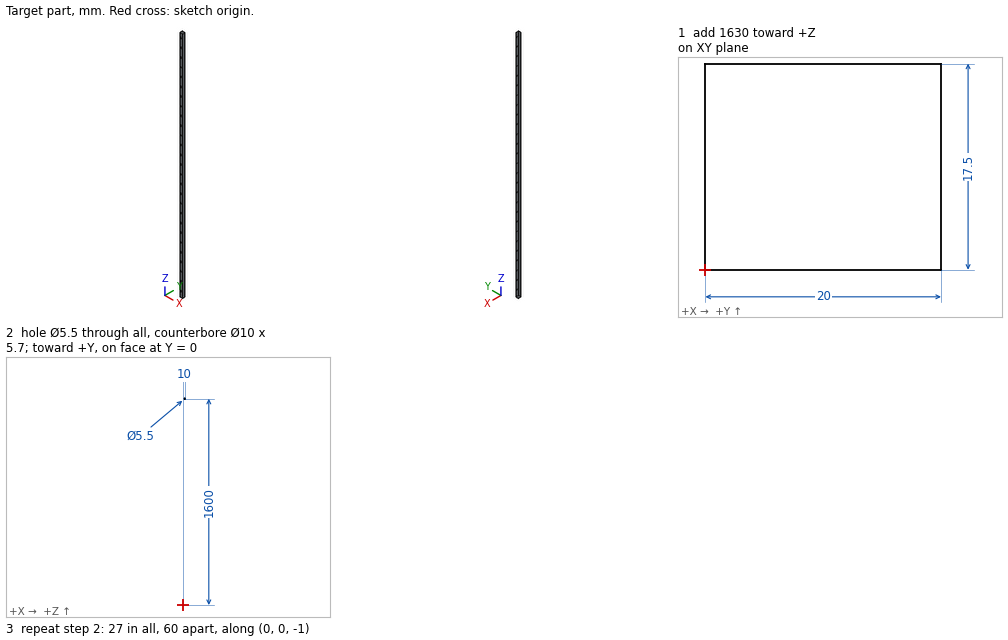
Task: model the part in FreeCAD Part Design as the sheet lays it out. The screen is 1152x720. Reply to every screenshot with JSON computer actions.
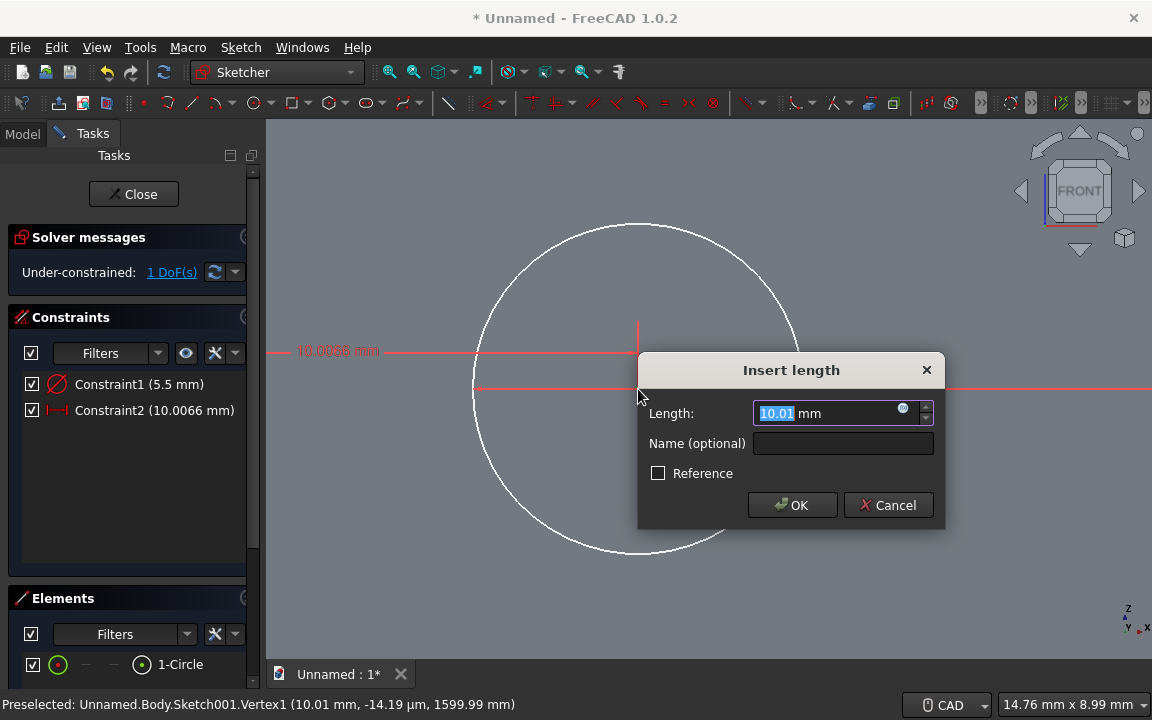
{"action": "type", "text": "10"}
{"action": "key", "text": "Return"}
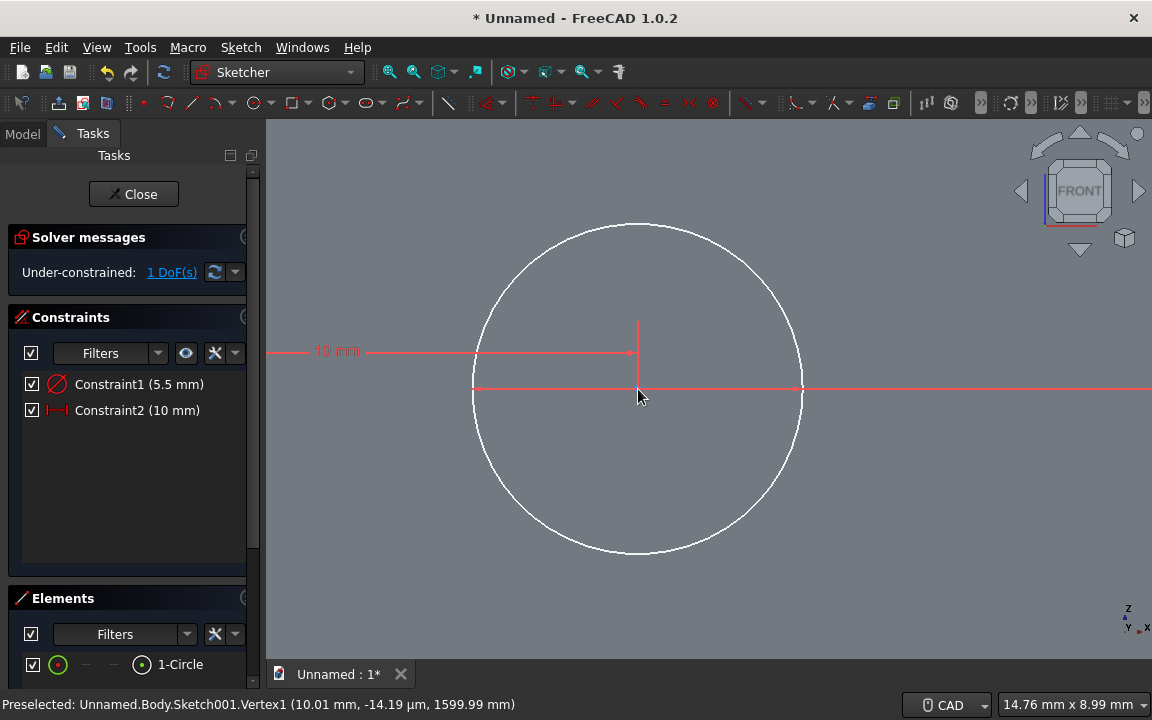
{"action": "left_click", "coordinate": [638, 389]}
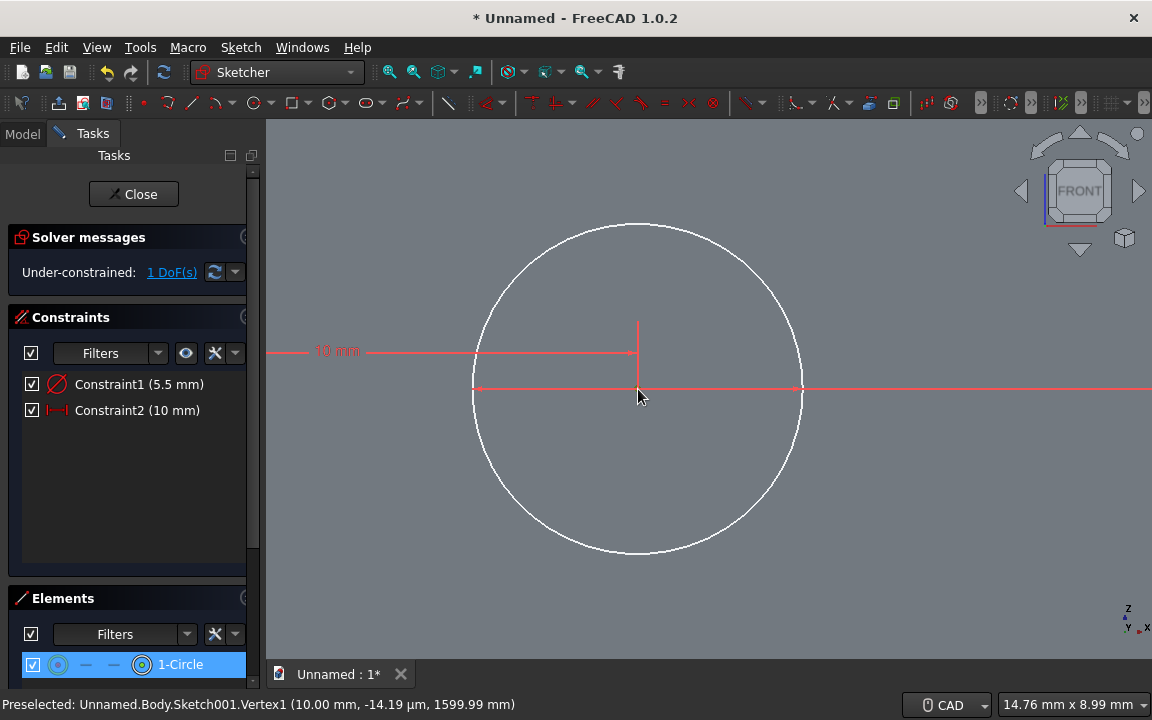
{"action": "left_click", "coordinate": [504, 104]}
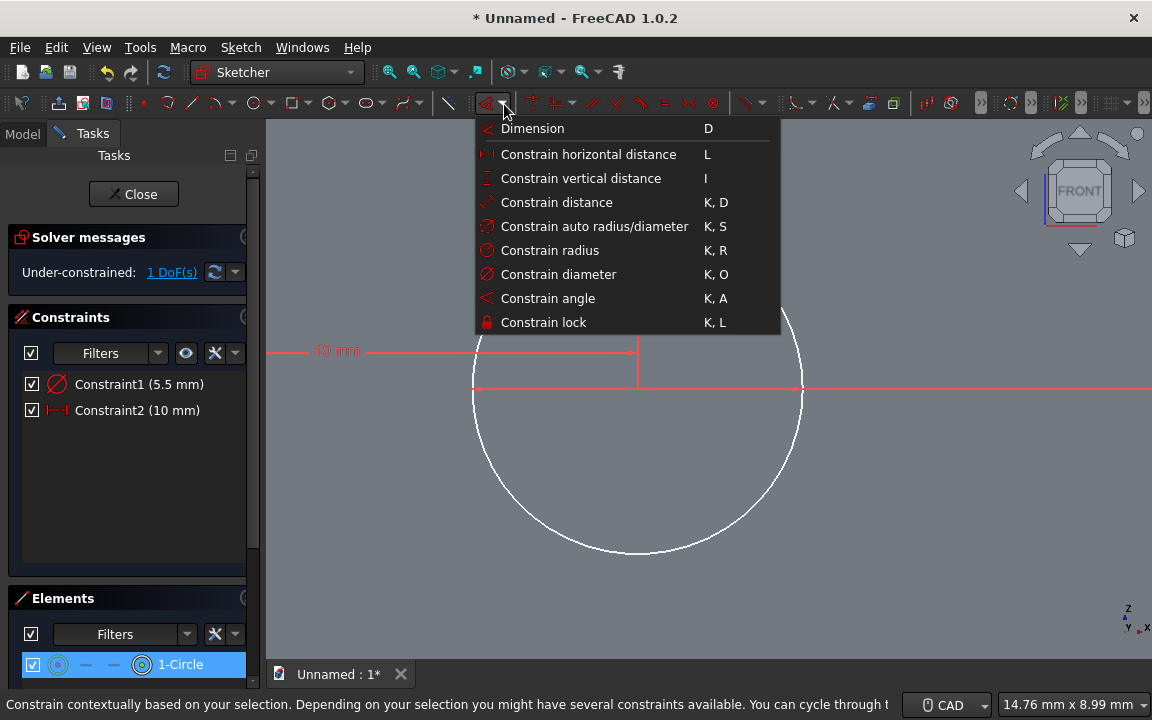
{"action": "left_click", "coordinate": [628, 178]}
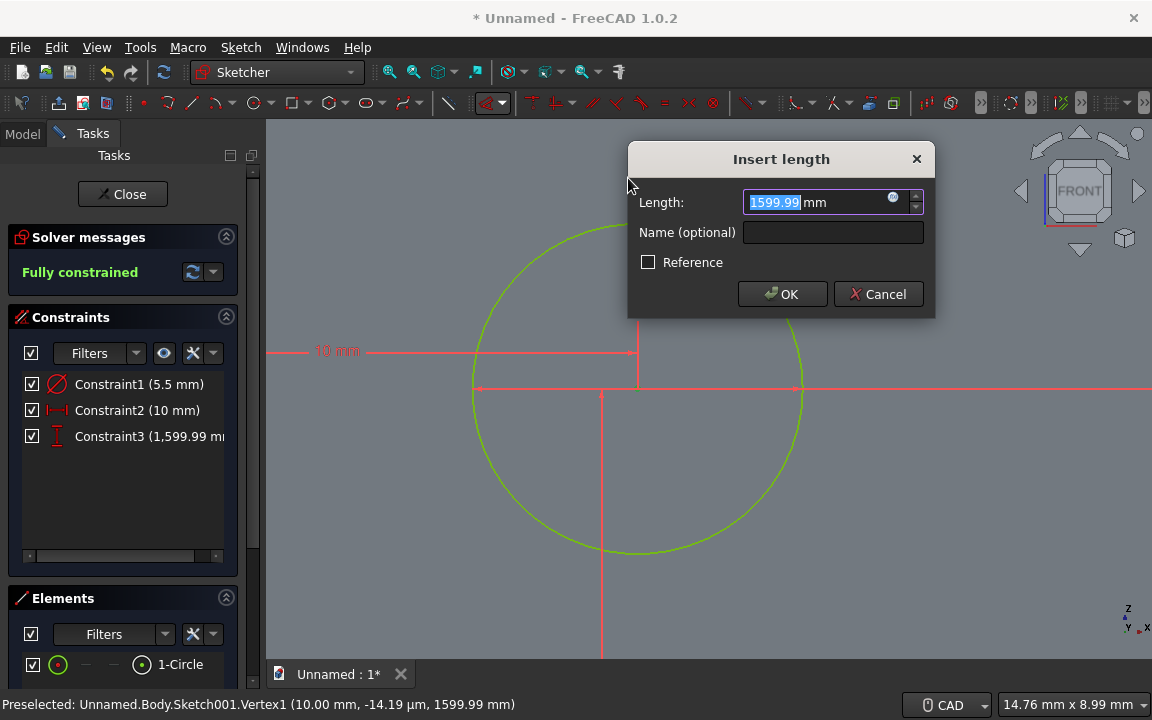
{"action": "type", "text": "1600"}
{"action": "key", "text": "Return"}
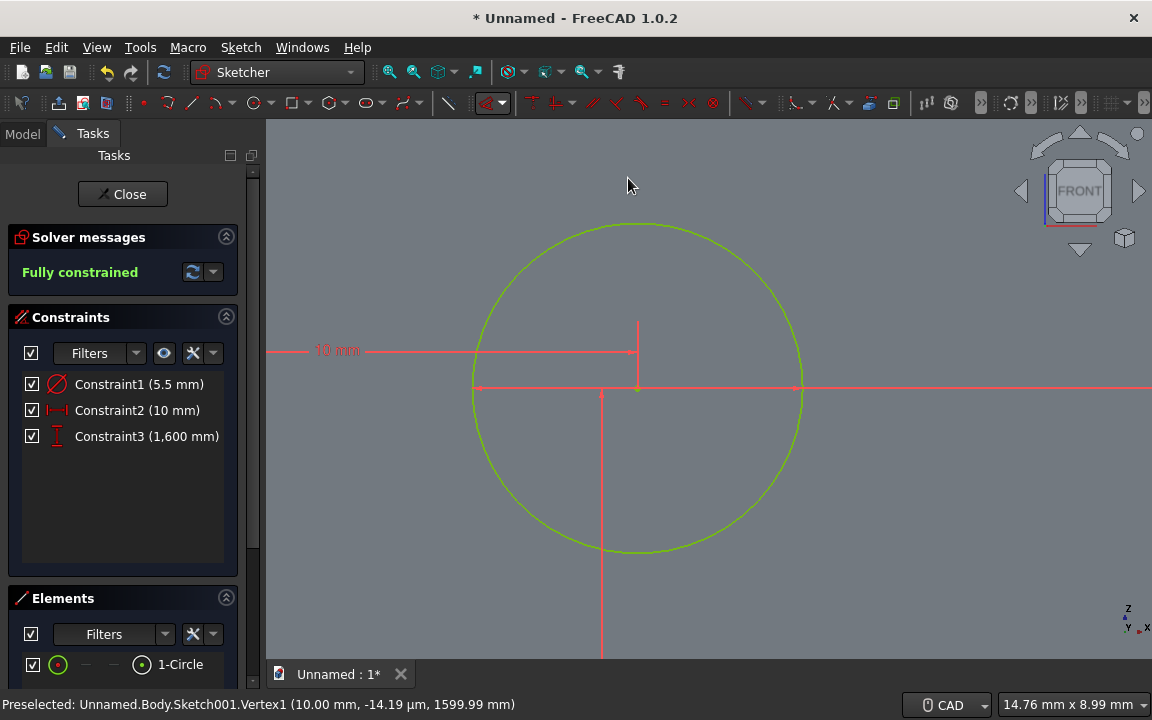
{"action": "left_click", "coordinate": [123, 194]}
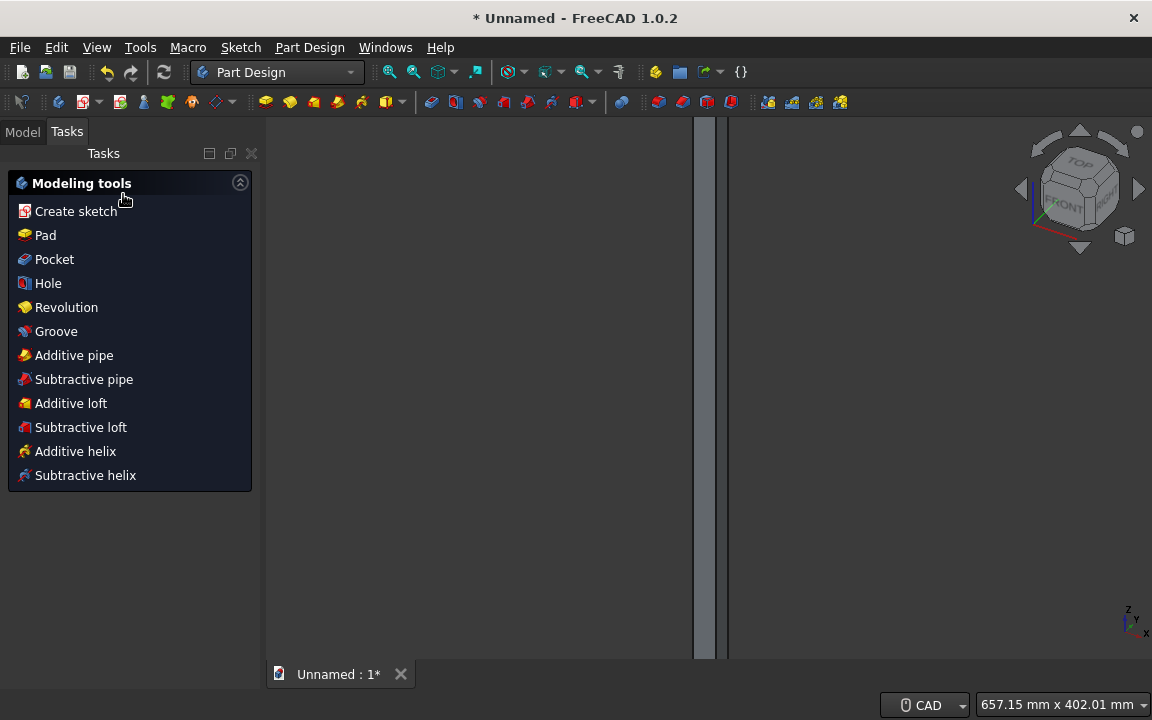
{"action": "left_click", "coordinate": [456, 102]}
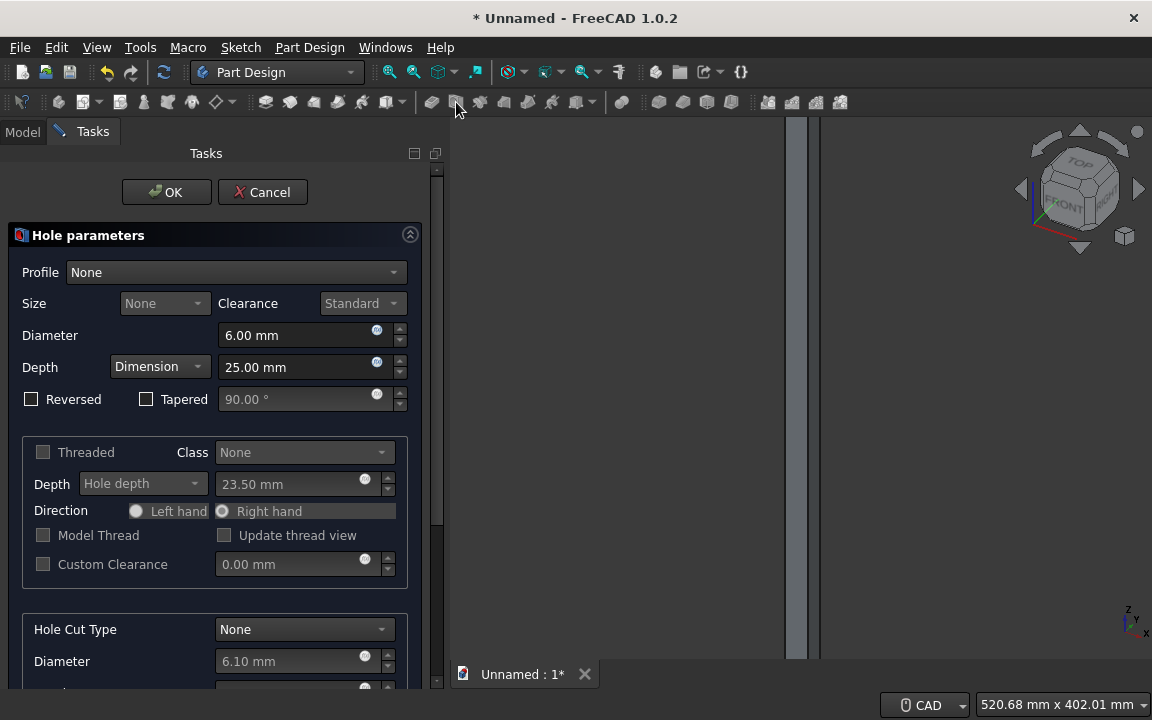
{"action": "triple_click", "coordinate": [305, 335]}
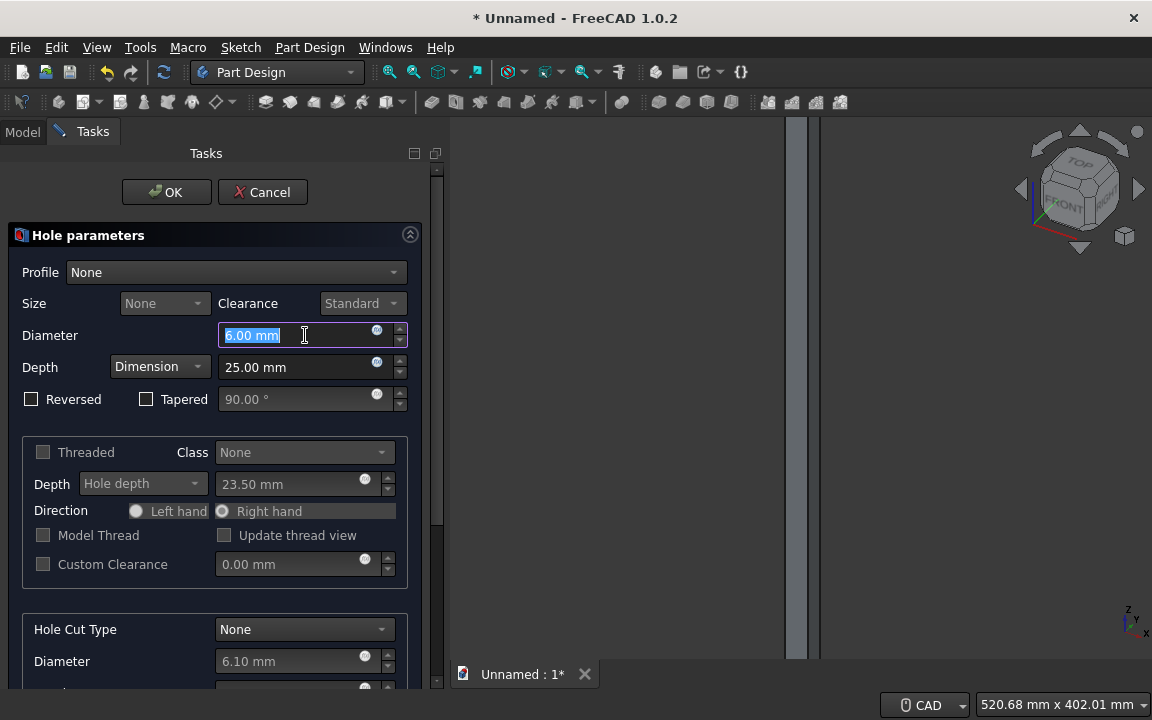
{"action": "type", "text": "5.5"}
{"action": "key", "text": "Tab"}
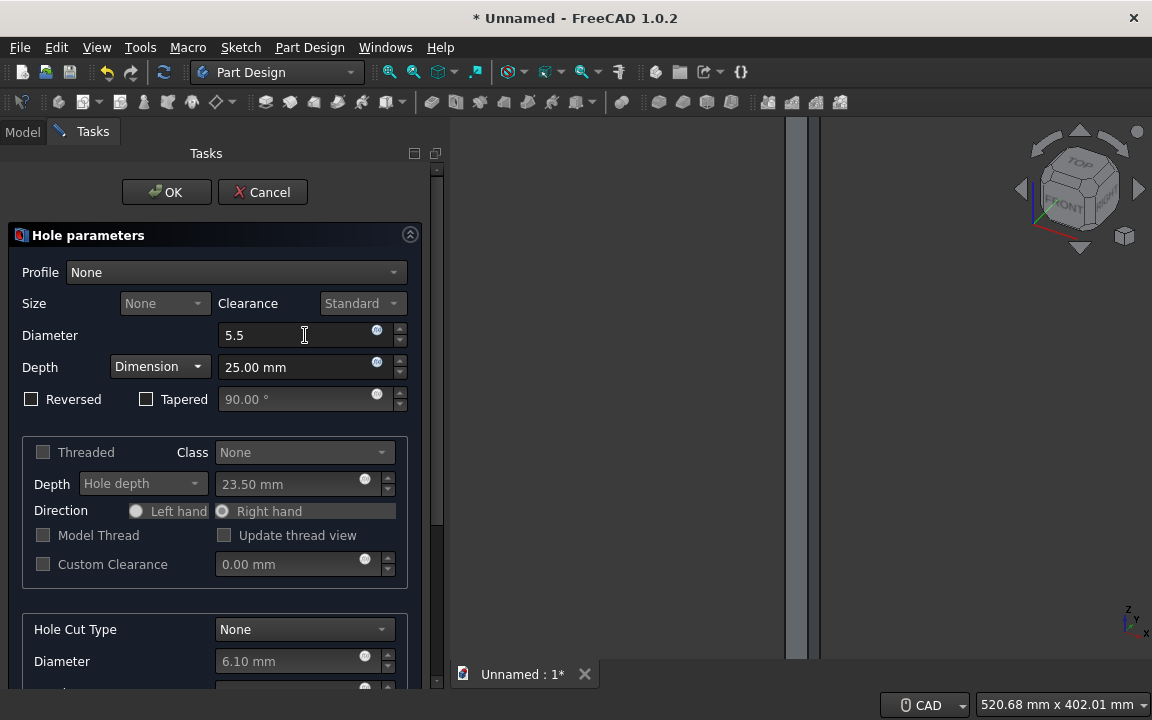
{"action": "left_click", "coordinate": [161, 366]}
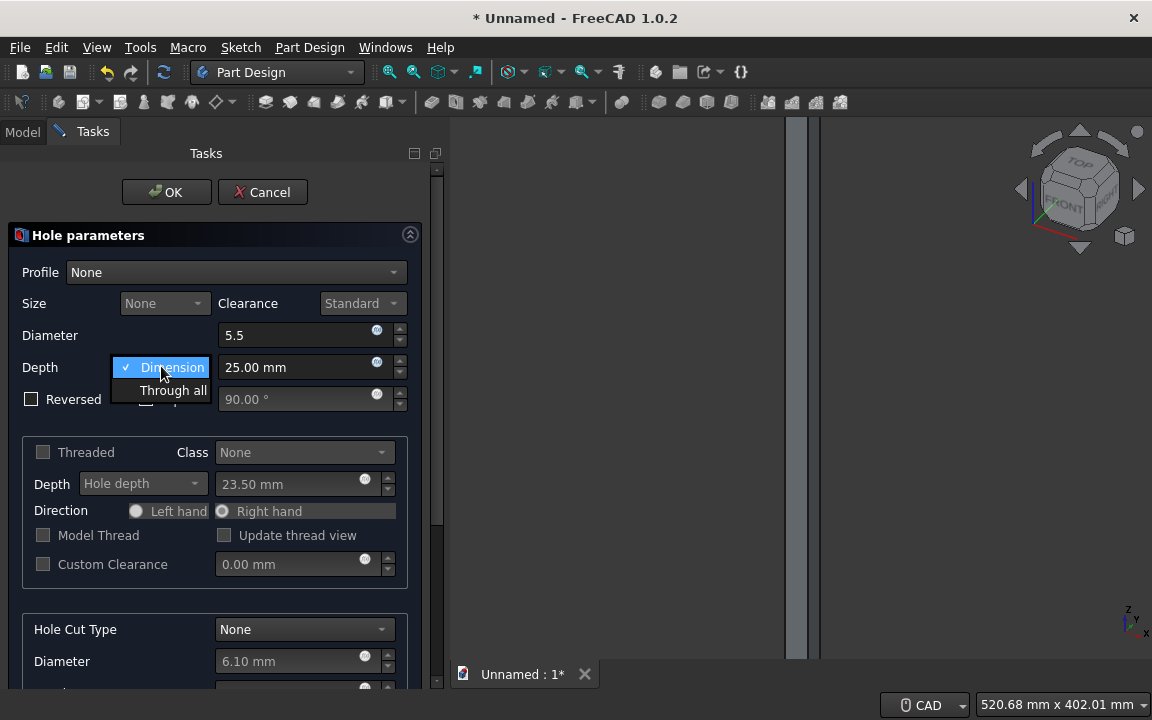
{"action": "left_click", "coordinate": [160, 390]}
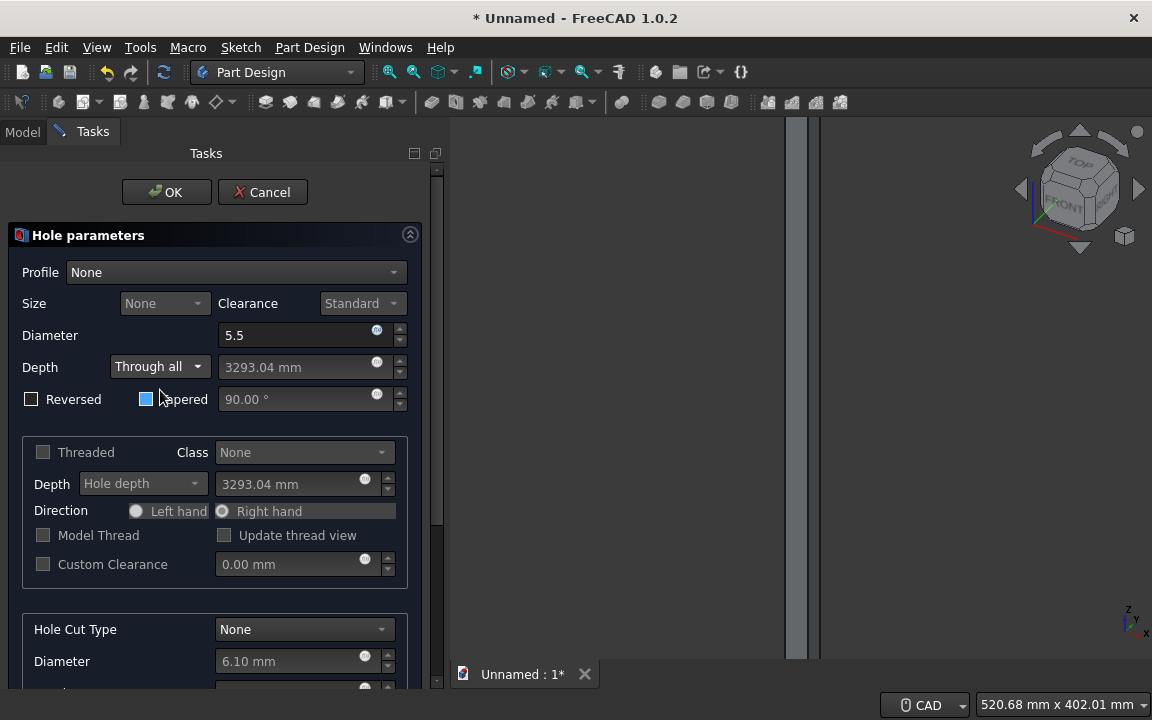
{"action": "left_click", "coordinate": [306, 630]}